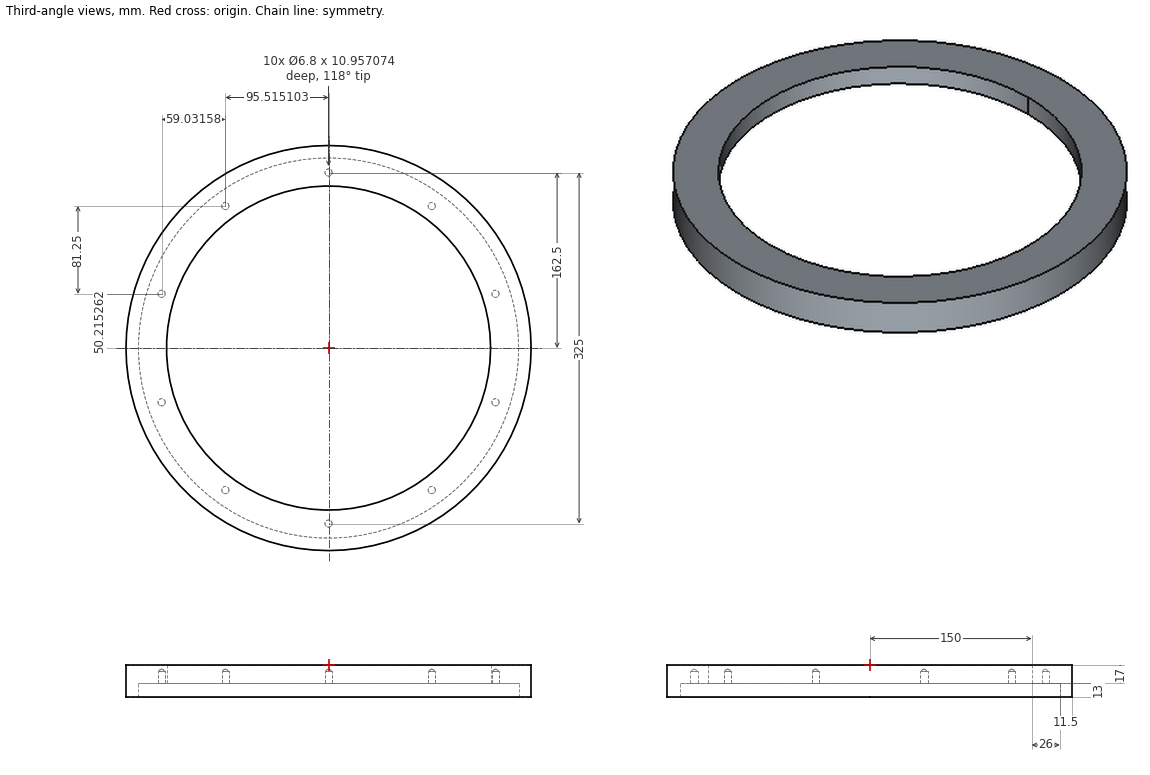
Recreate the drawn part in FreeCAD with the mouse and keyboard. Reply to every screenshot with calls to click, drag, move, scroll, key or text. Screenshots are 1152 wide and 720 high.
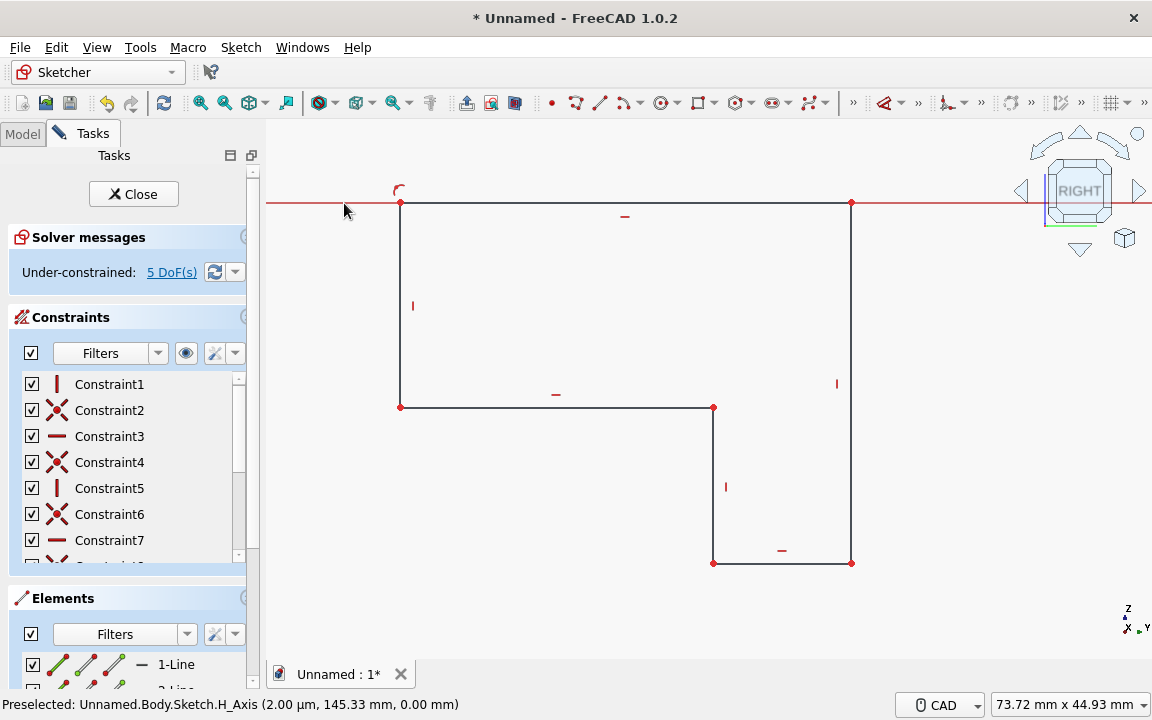
click(400, 264)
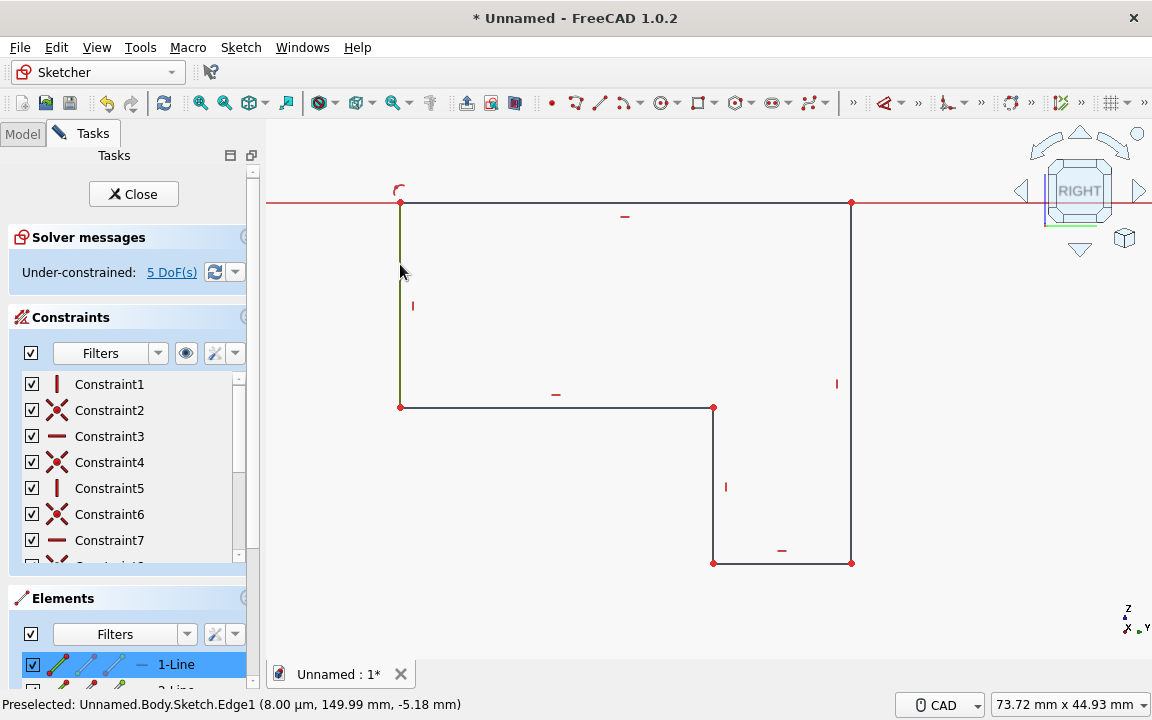
key(i)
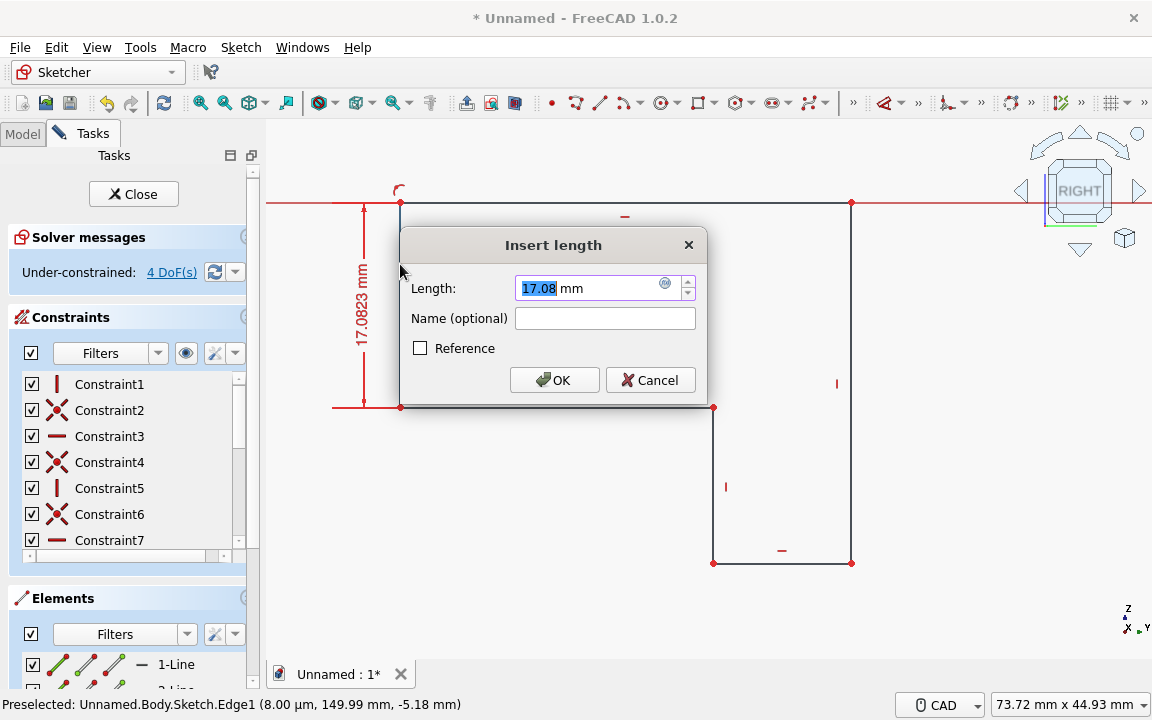
text(17)
key(Return)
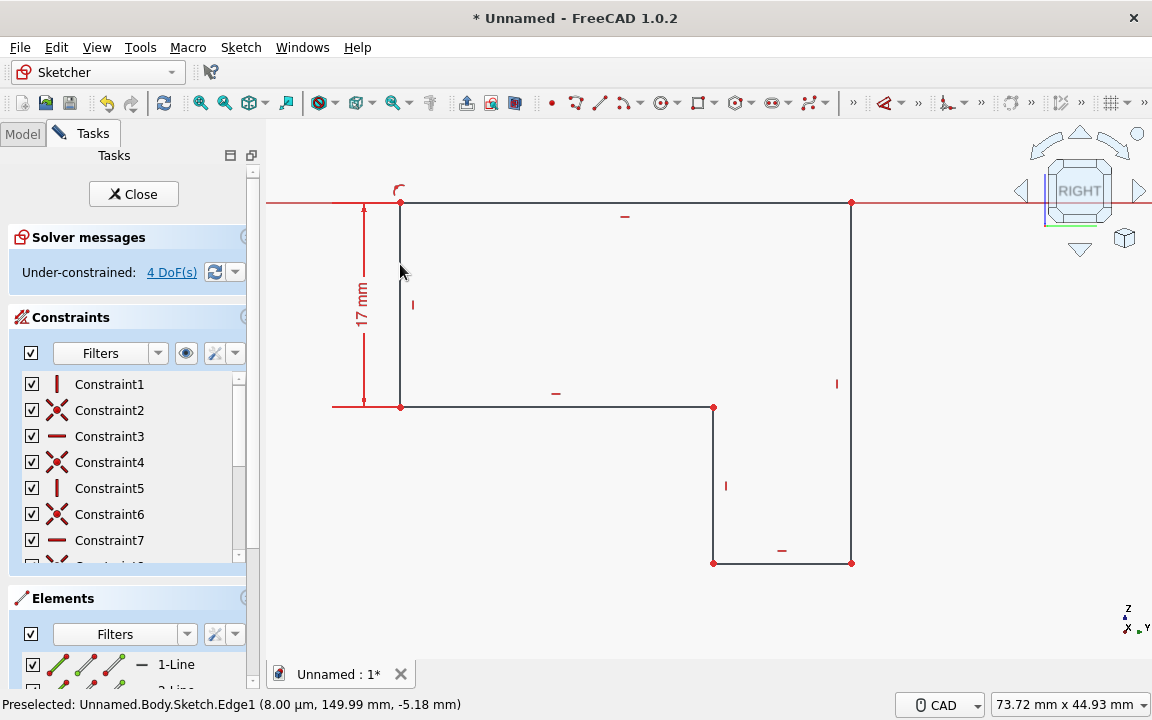
click(494, 407)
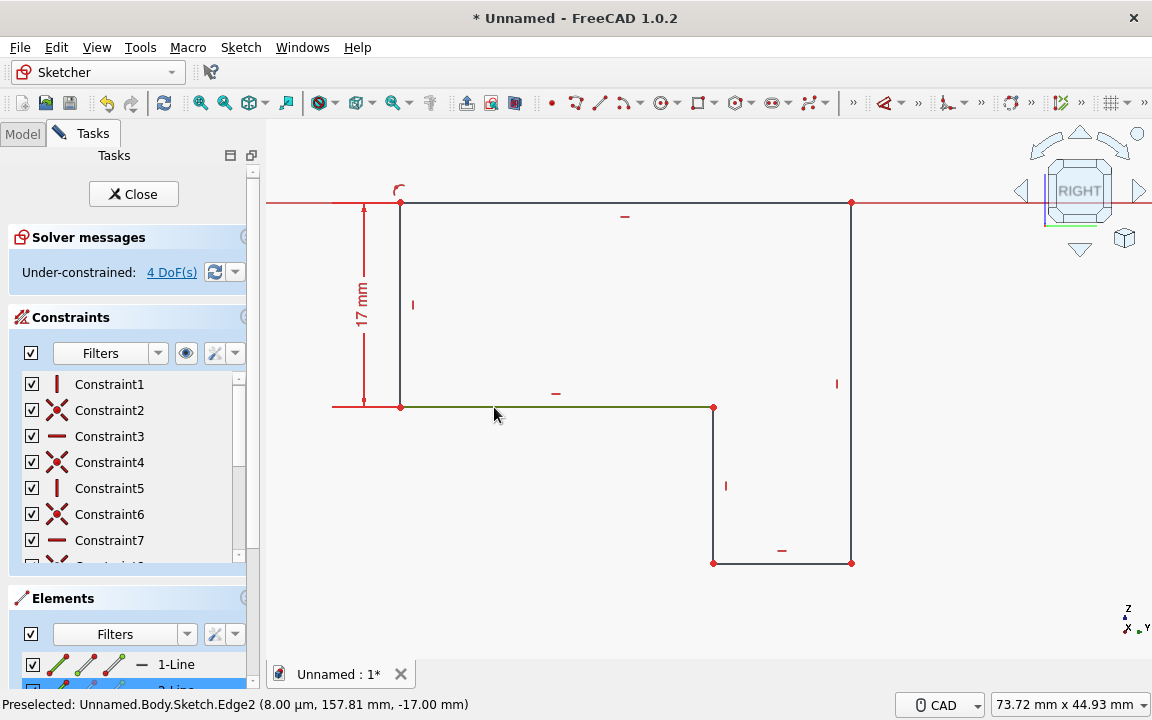
key(l)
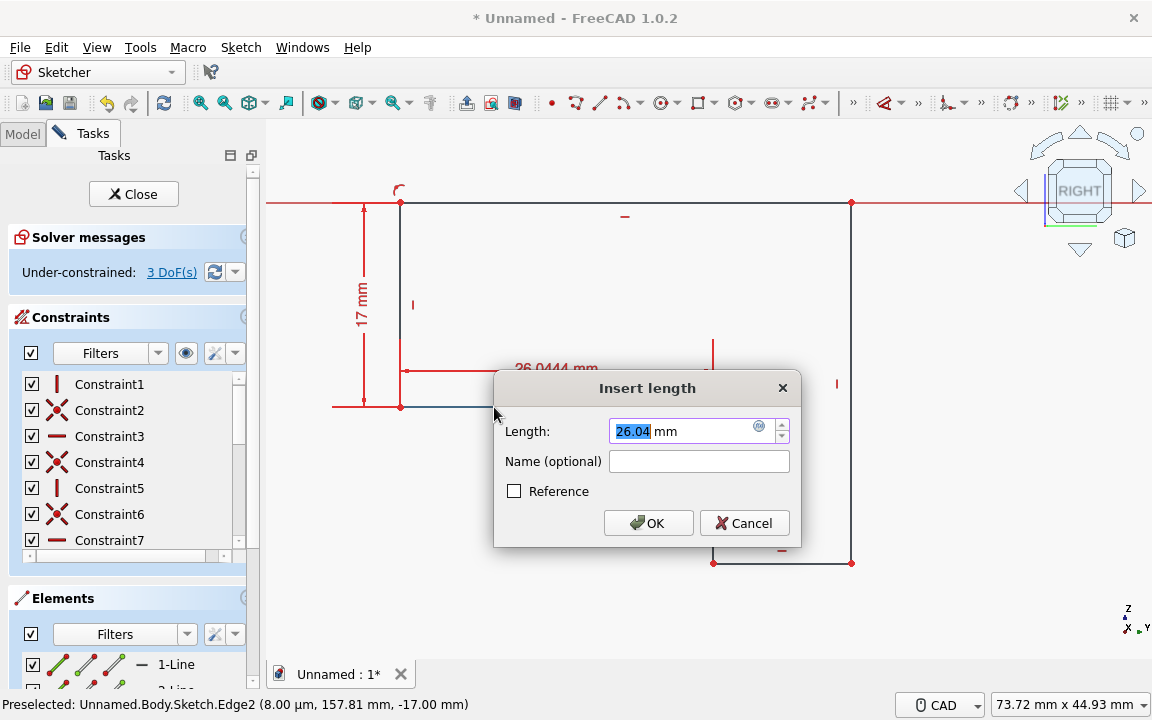
text(26)
key(Return)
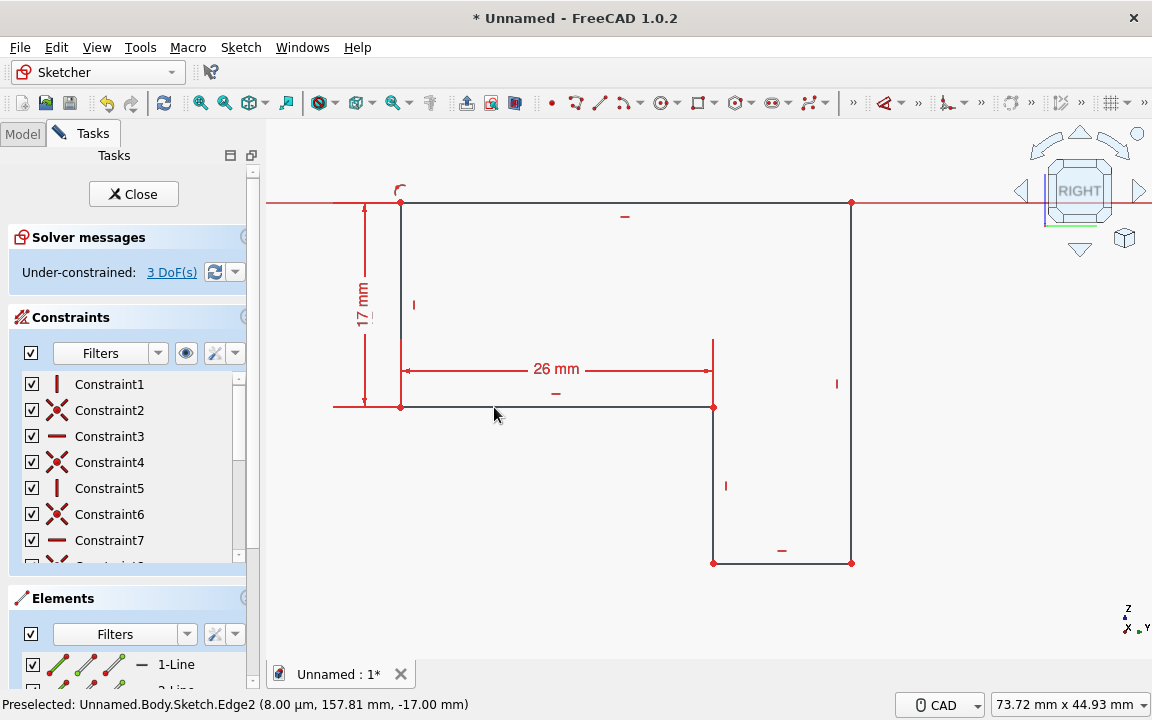
click(713, 454)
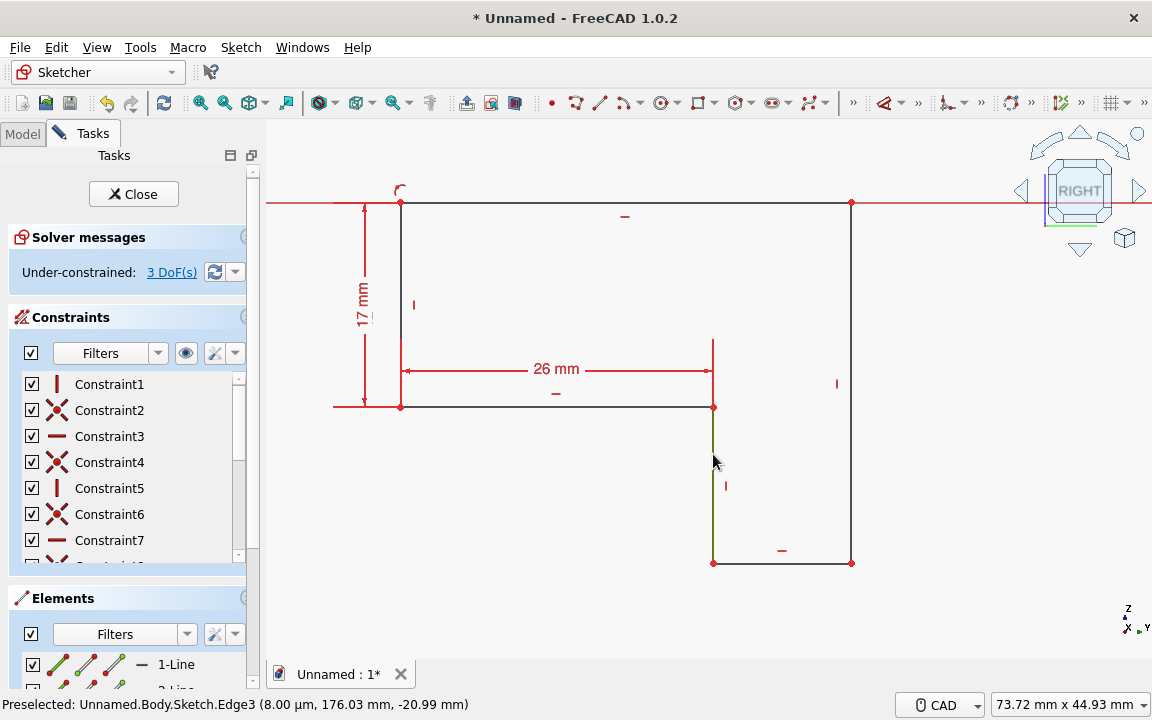
key(i)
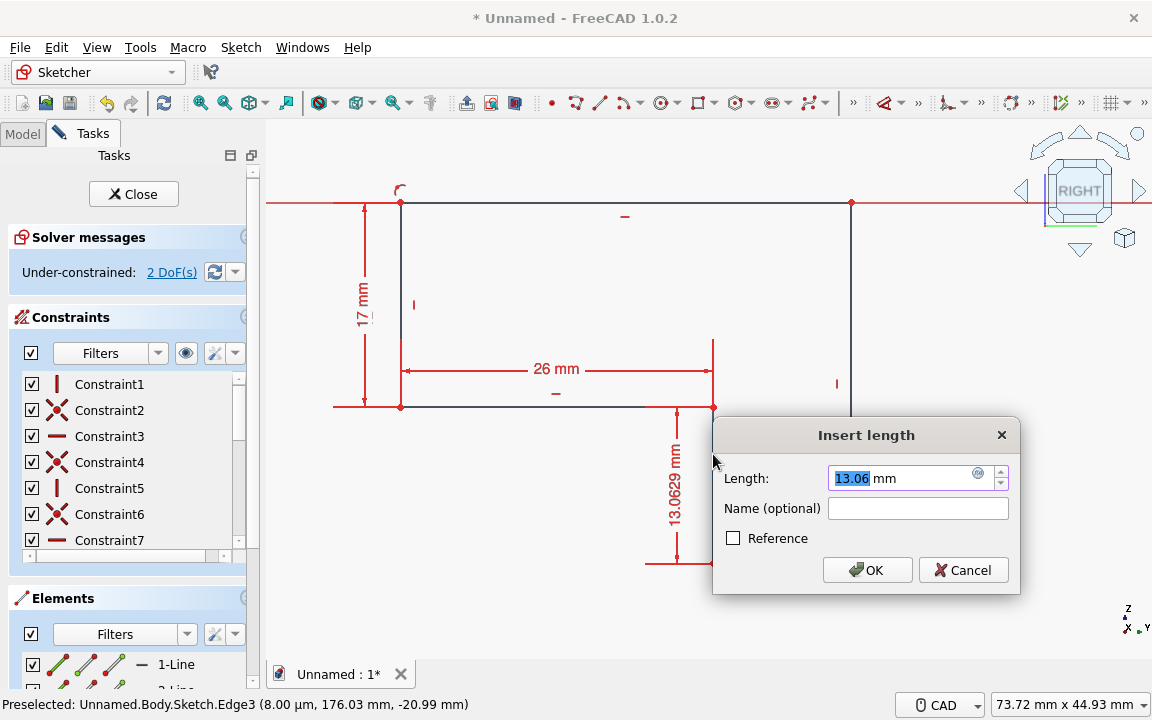
text(13)
key(Return)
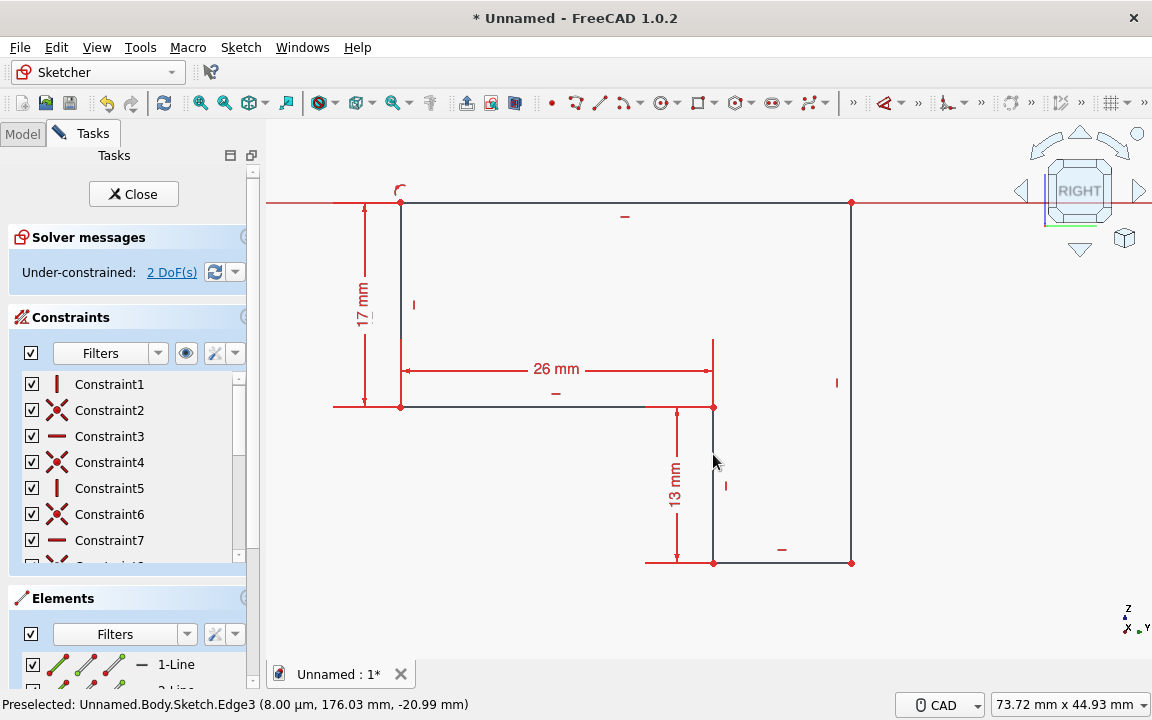
click(754, 563)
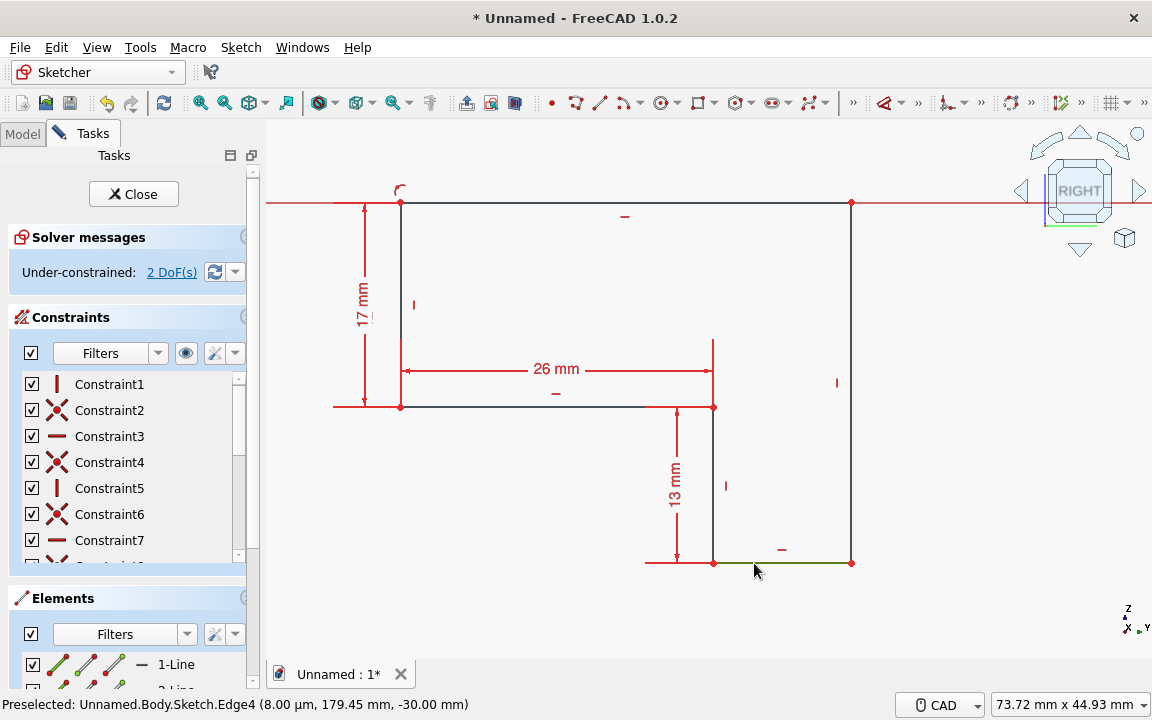
key(l)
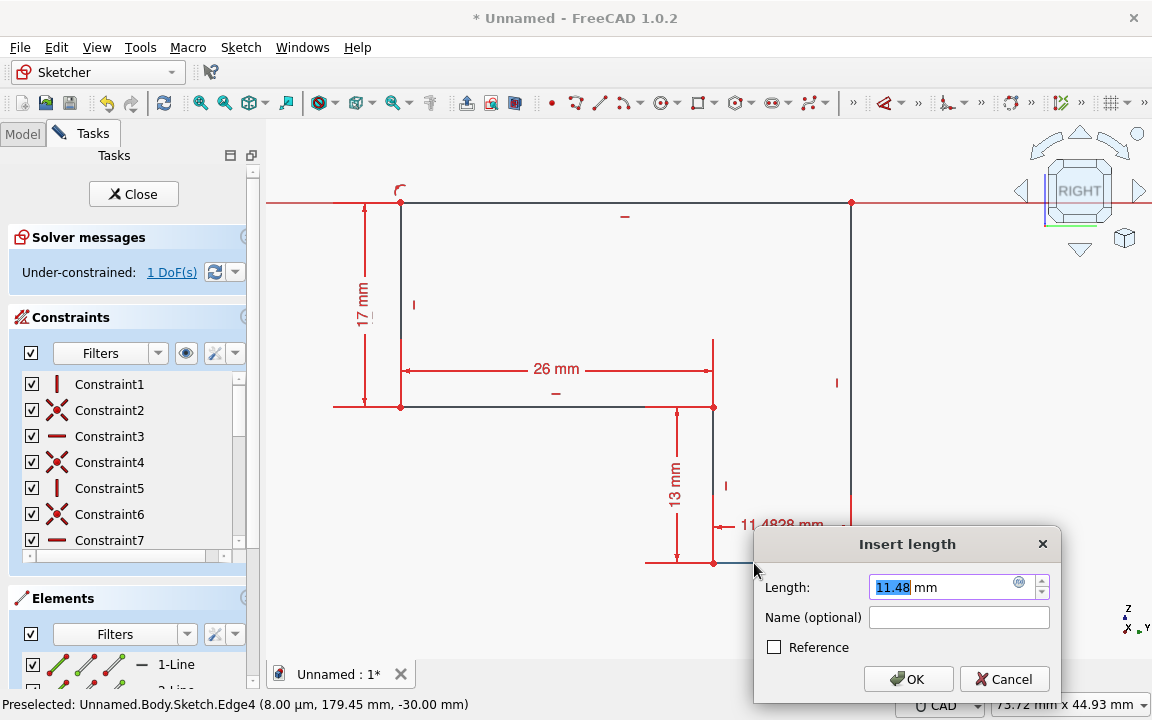
text(11.5)
key(Return)